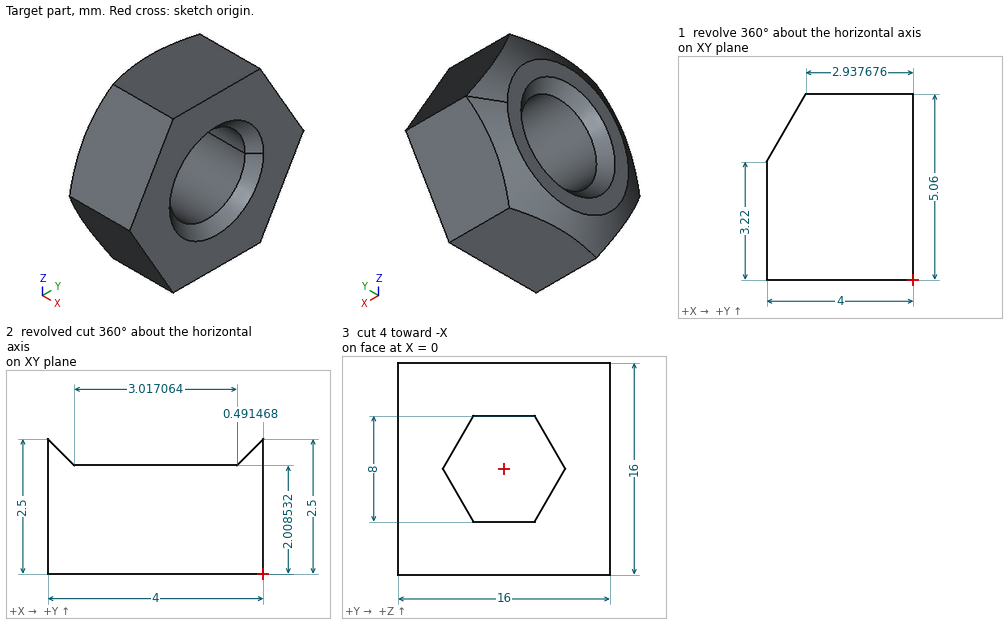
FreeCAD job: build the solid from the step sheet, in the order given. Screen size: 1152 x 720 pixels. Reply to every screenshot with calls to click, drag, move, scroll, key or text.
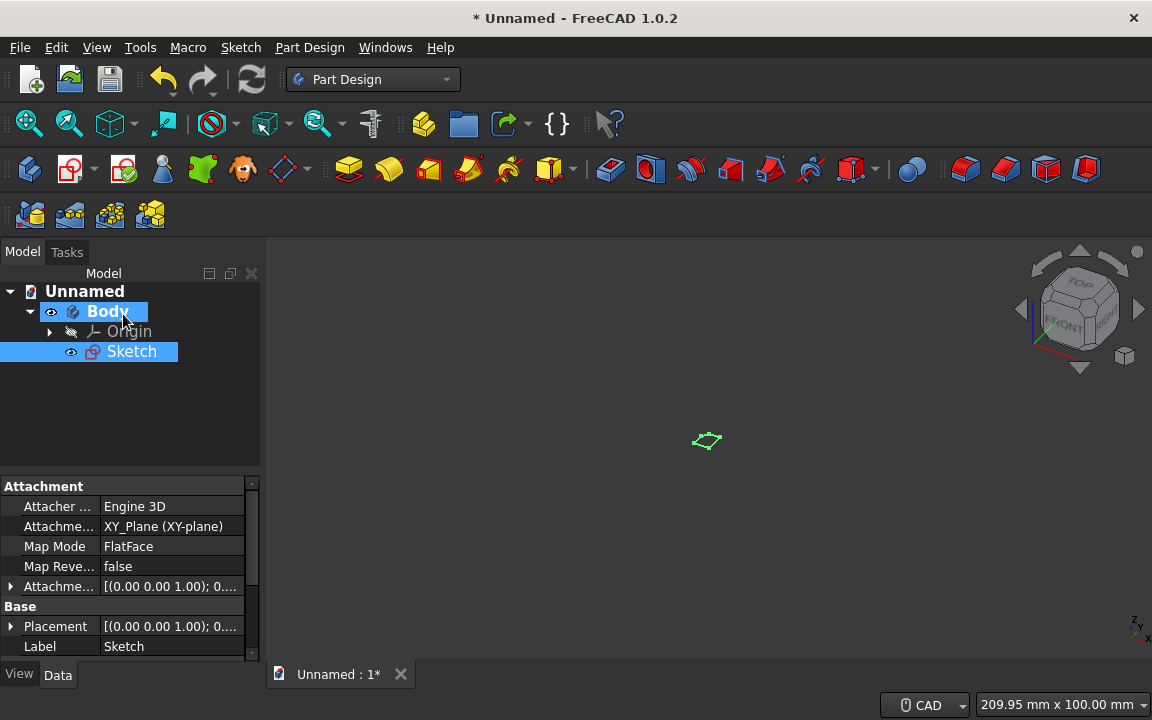
click(390, 170)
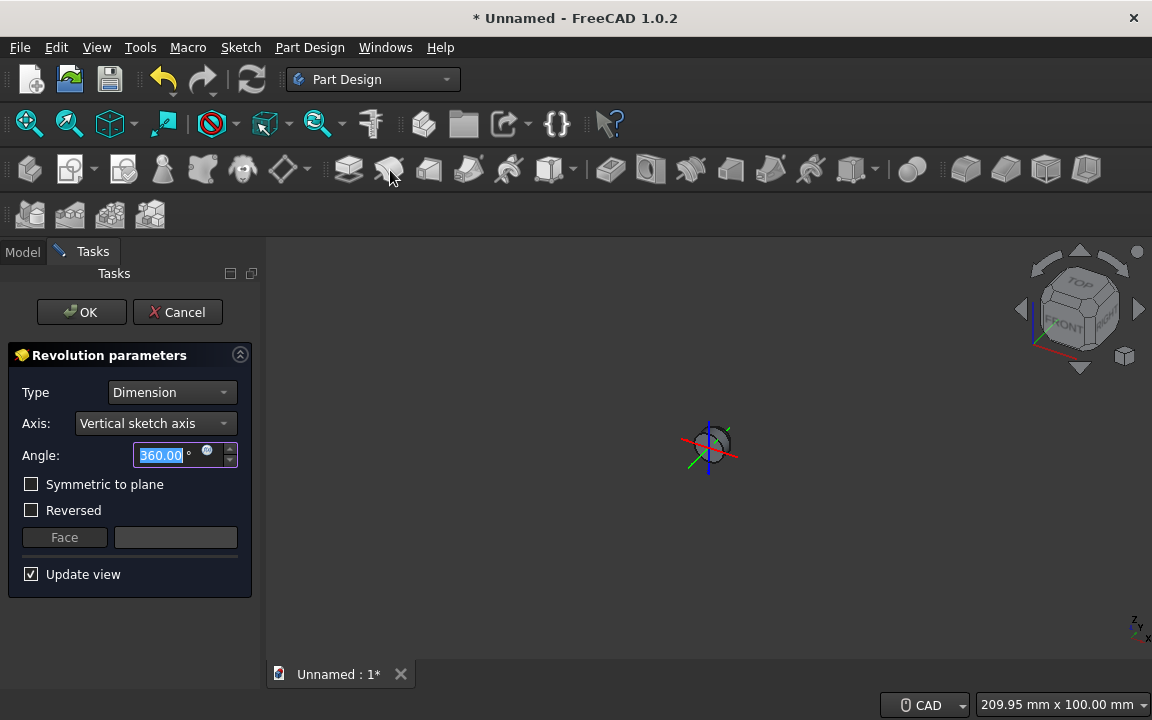
click(156, 424)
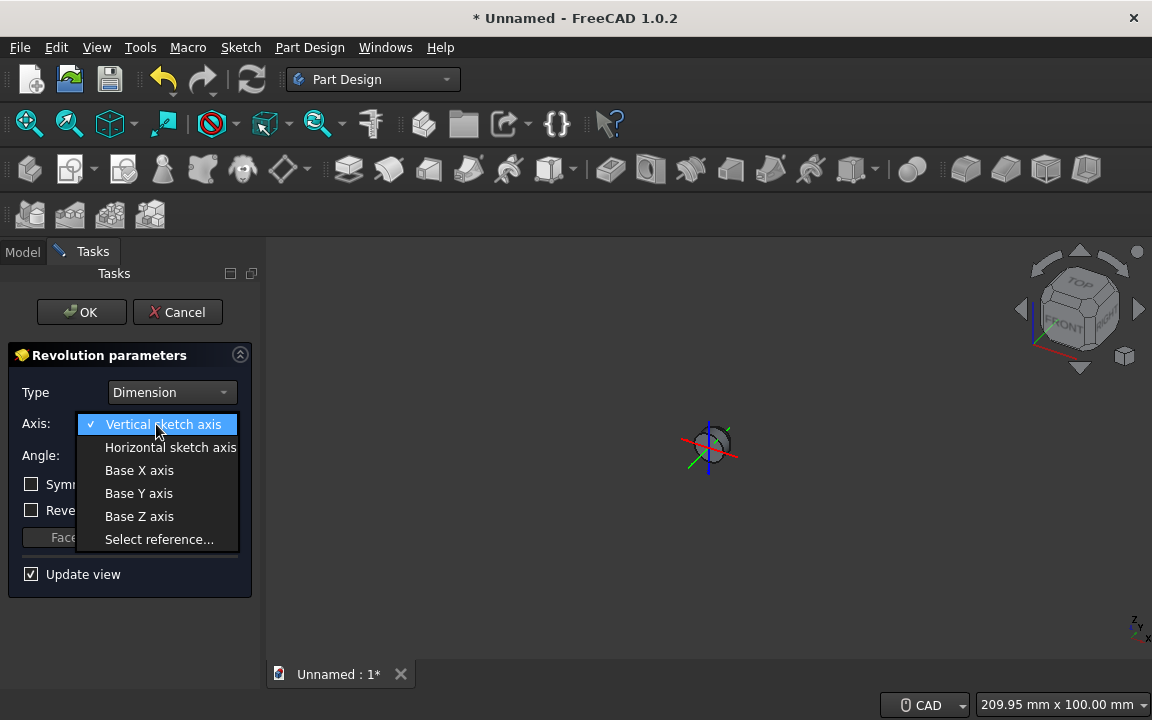
click(156, 448)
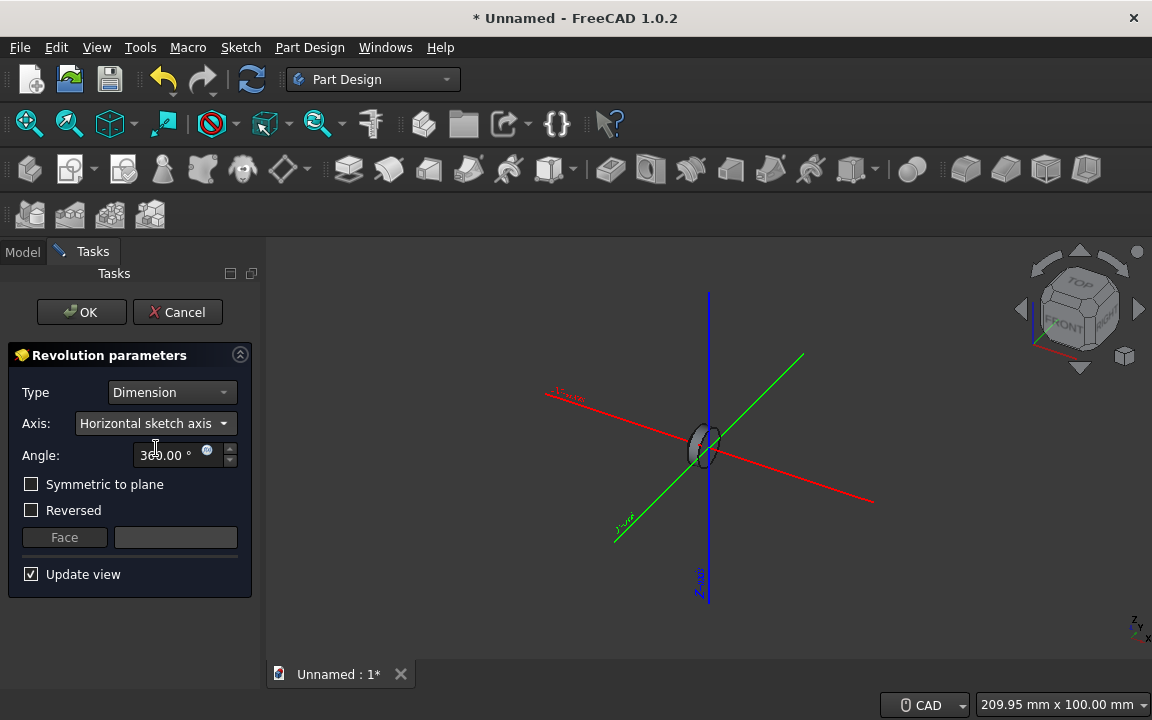
click(82, 312)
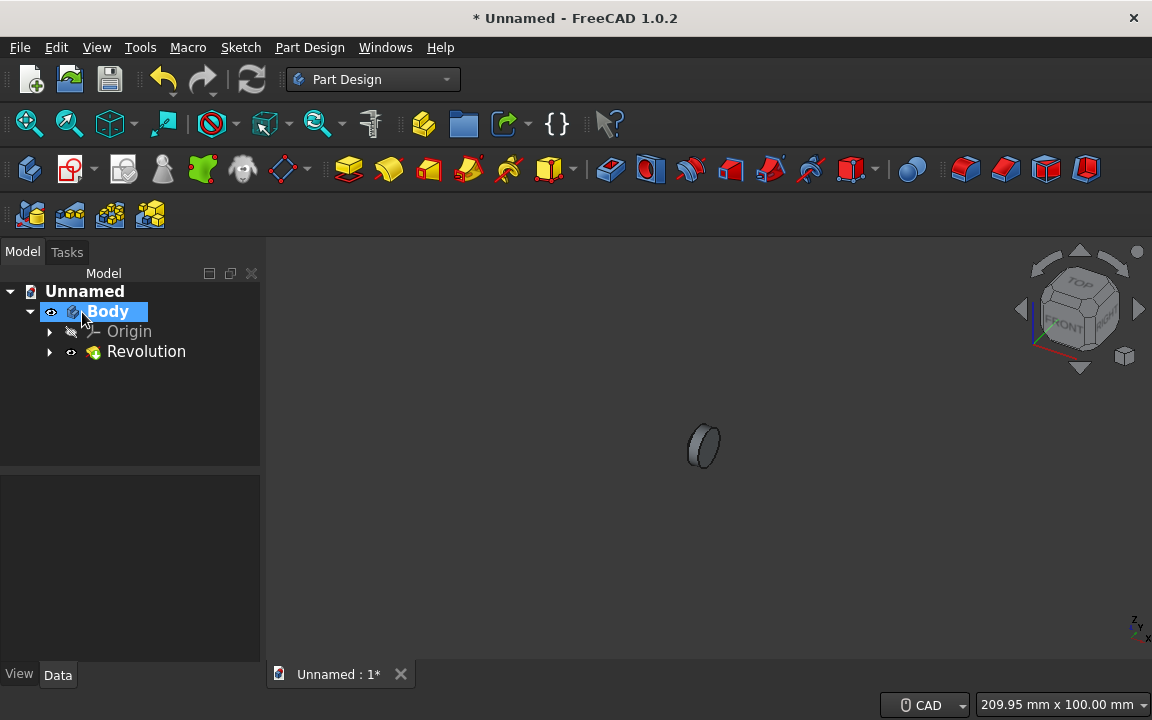
key(v)
key(f)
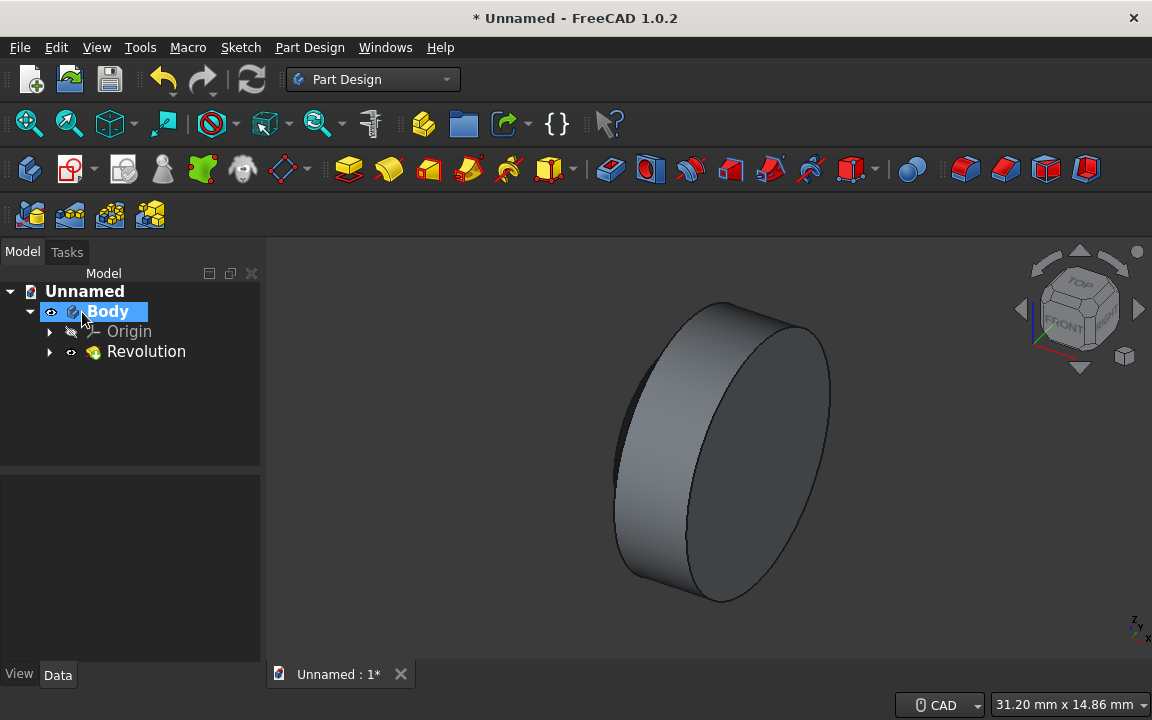
click(70, 170)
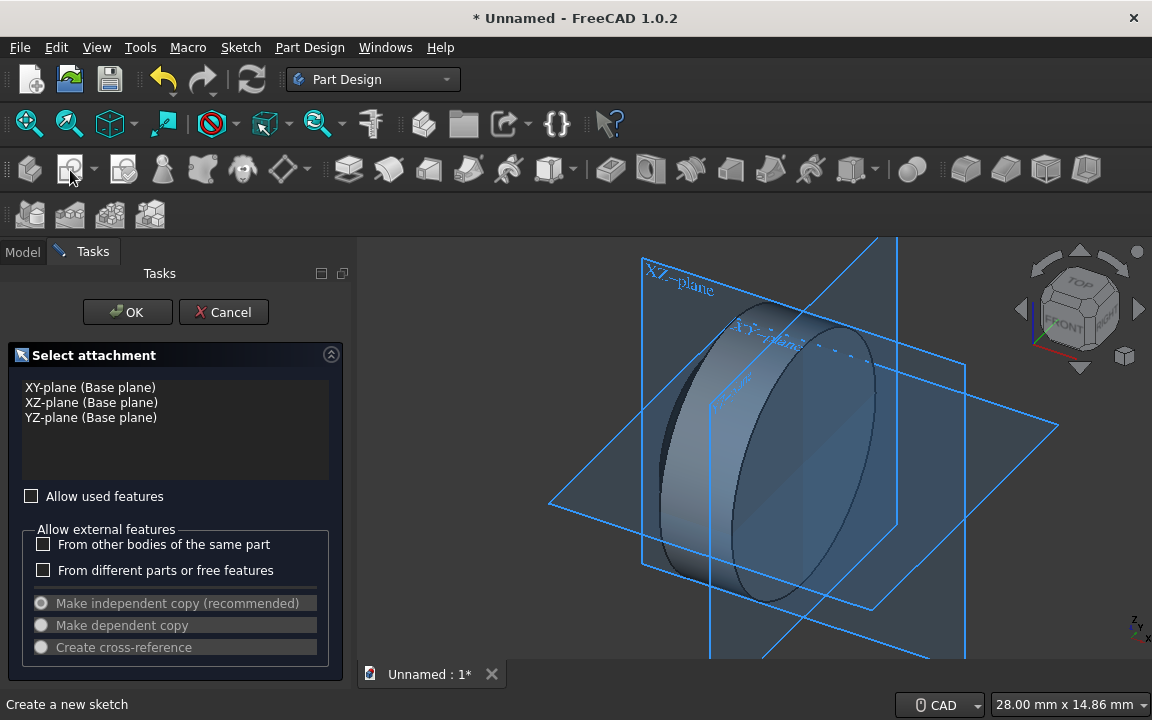
click(82, 388)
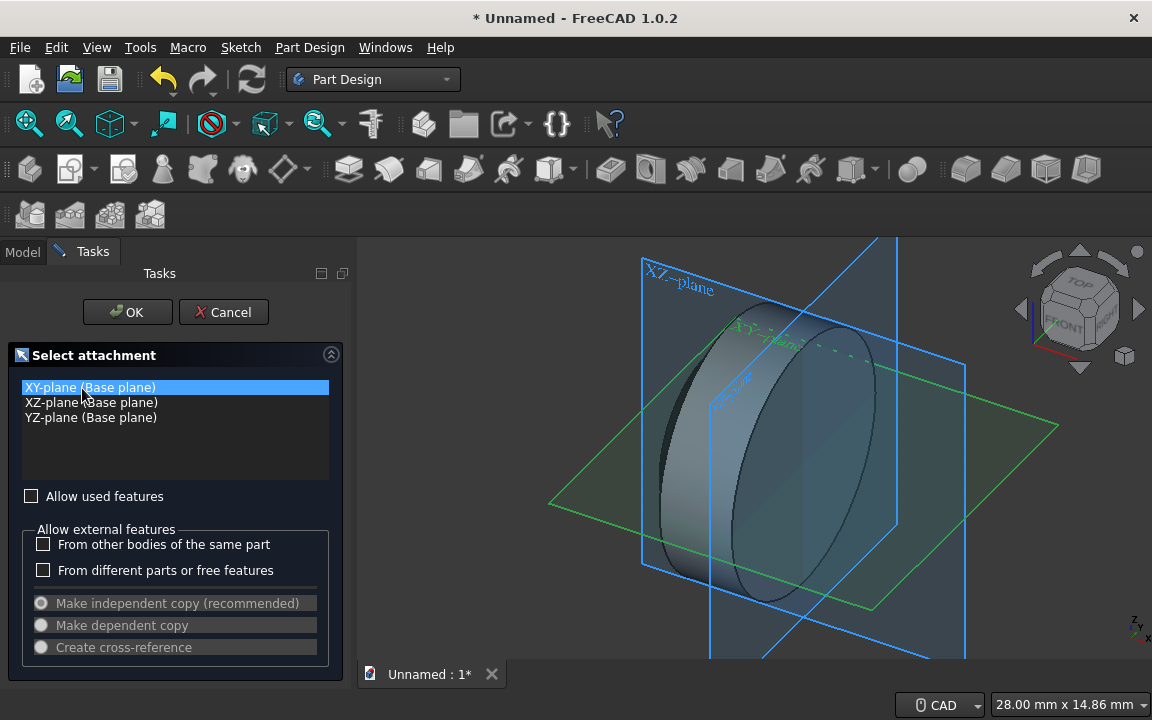
click(128, 312)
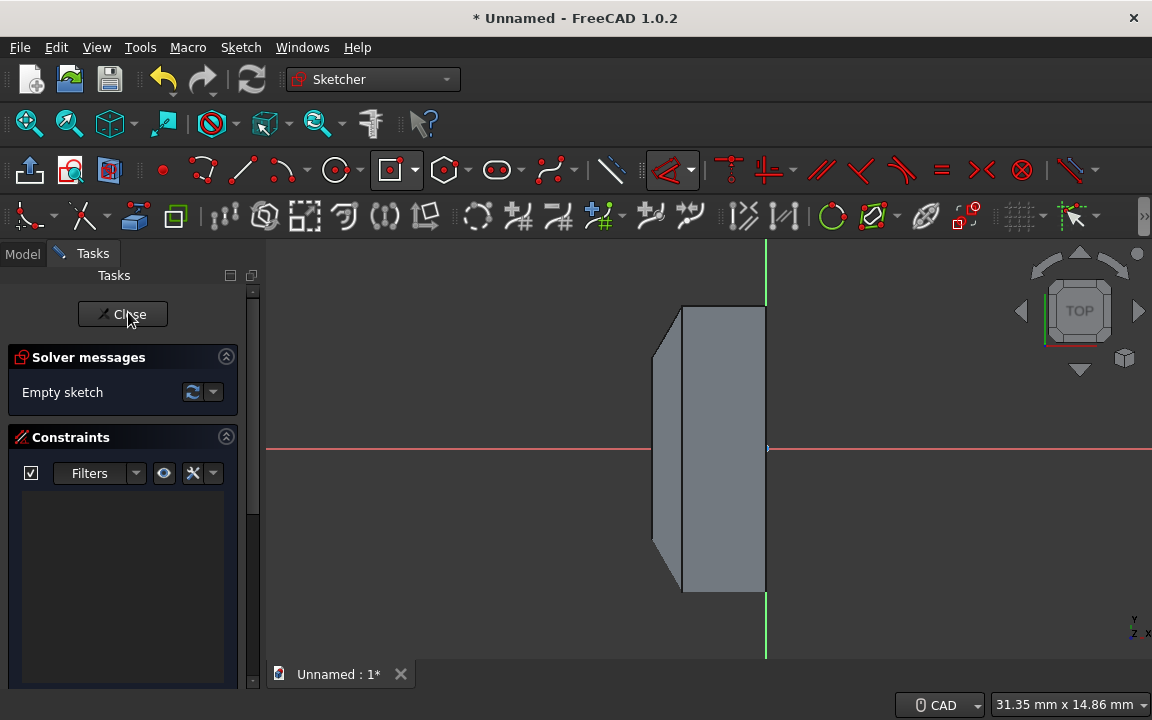
key(q)
key(s)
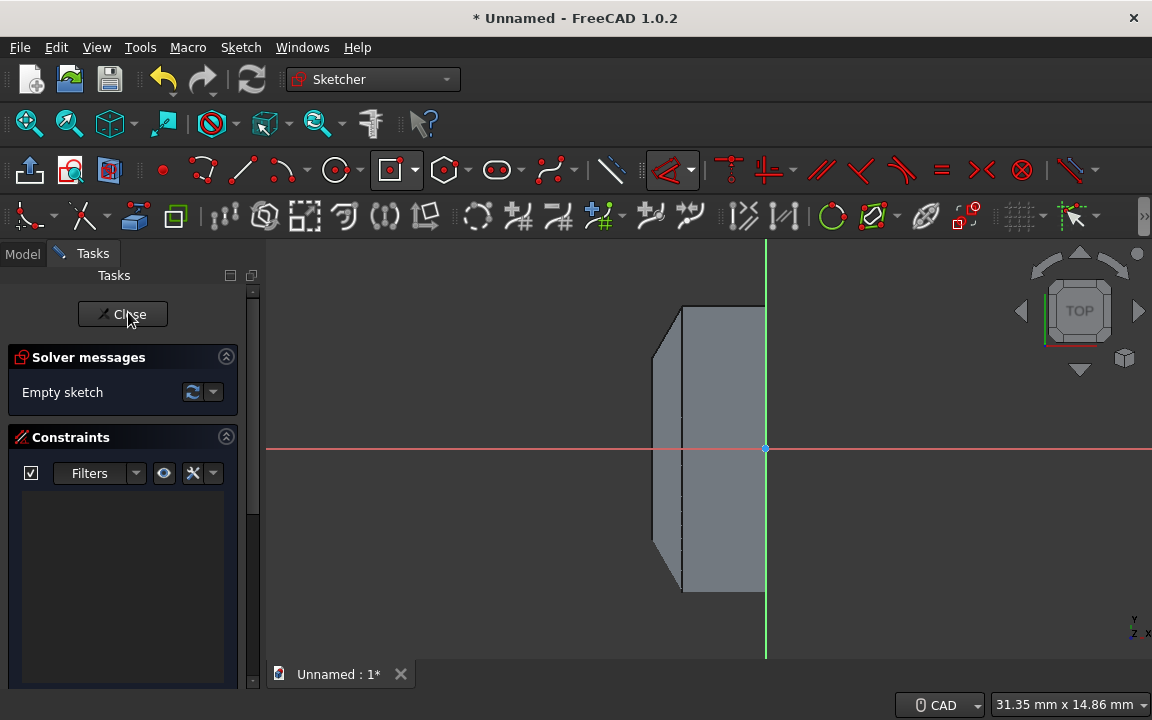
scroll(739, 398, up, 6)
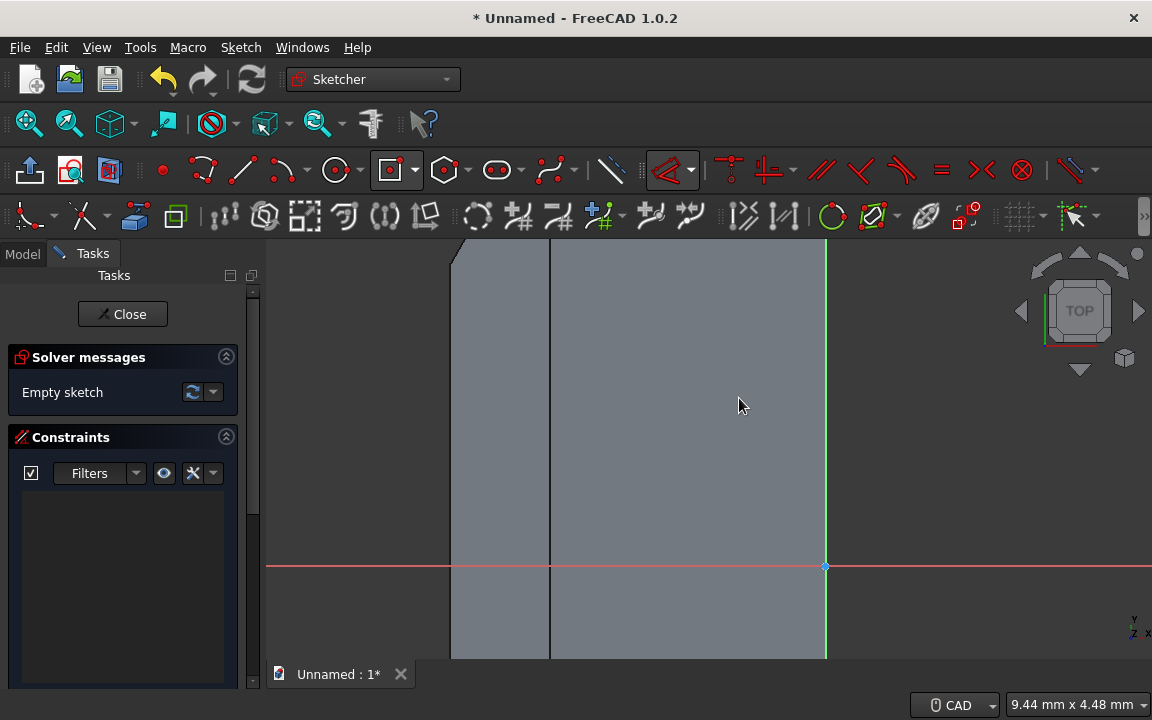
key(g)
key(m)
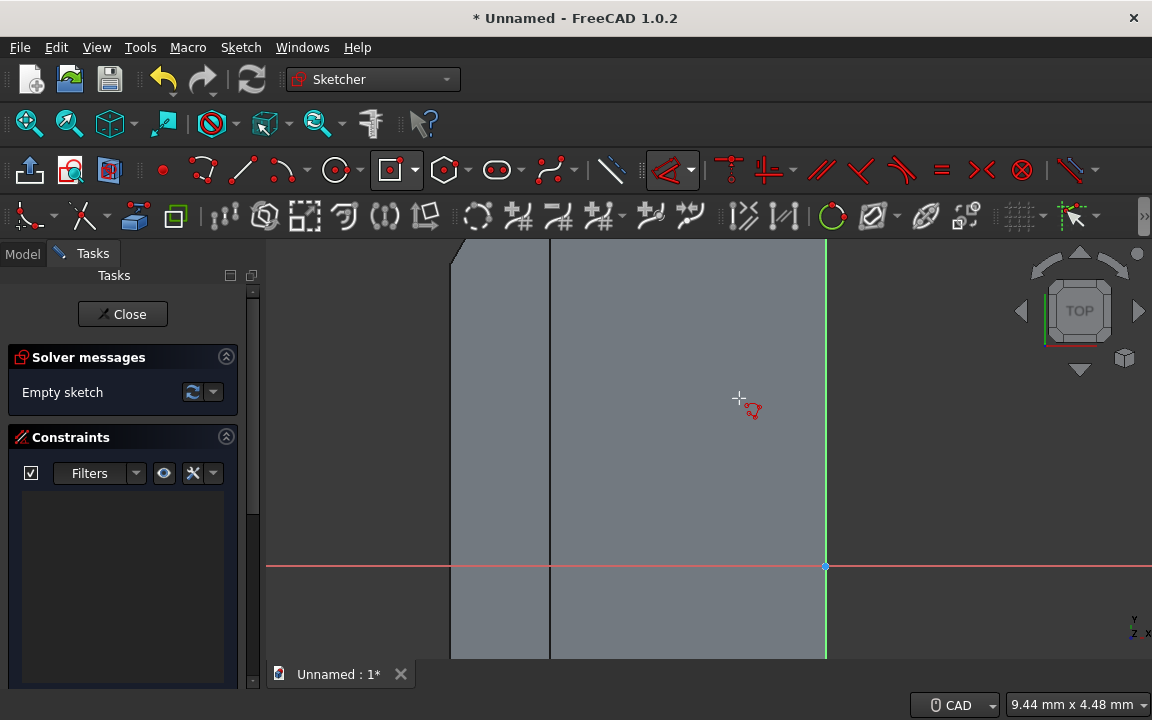
click(826, 566)
click(817, 332)
click(780, 378)
click(497, 378)
click(450, 332)
click(450, 557)
click(826, 566)
key(Escape)
key(Escape)